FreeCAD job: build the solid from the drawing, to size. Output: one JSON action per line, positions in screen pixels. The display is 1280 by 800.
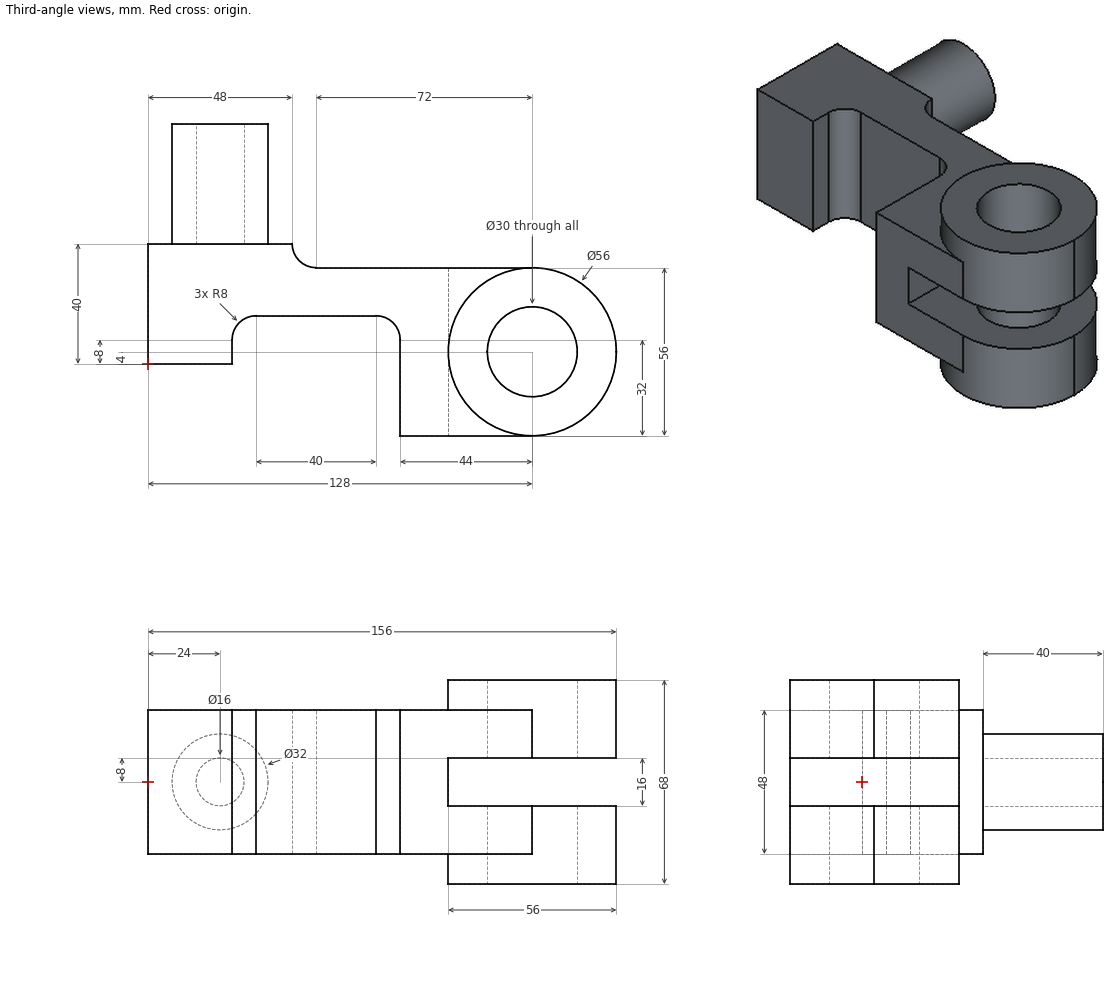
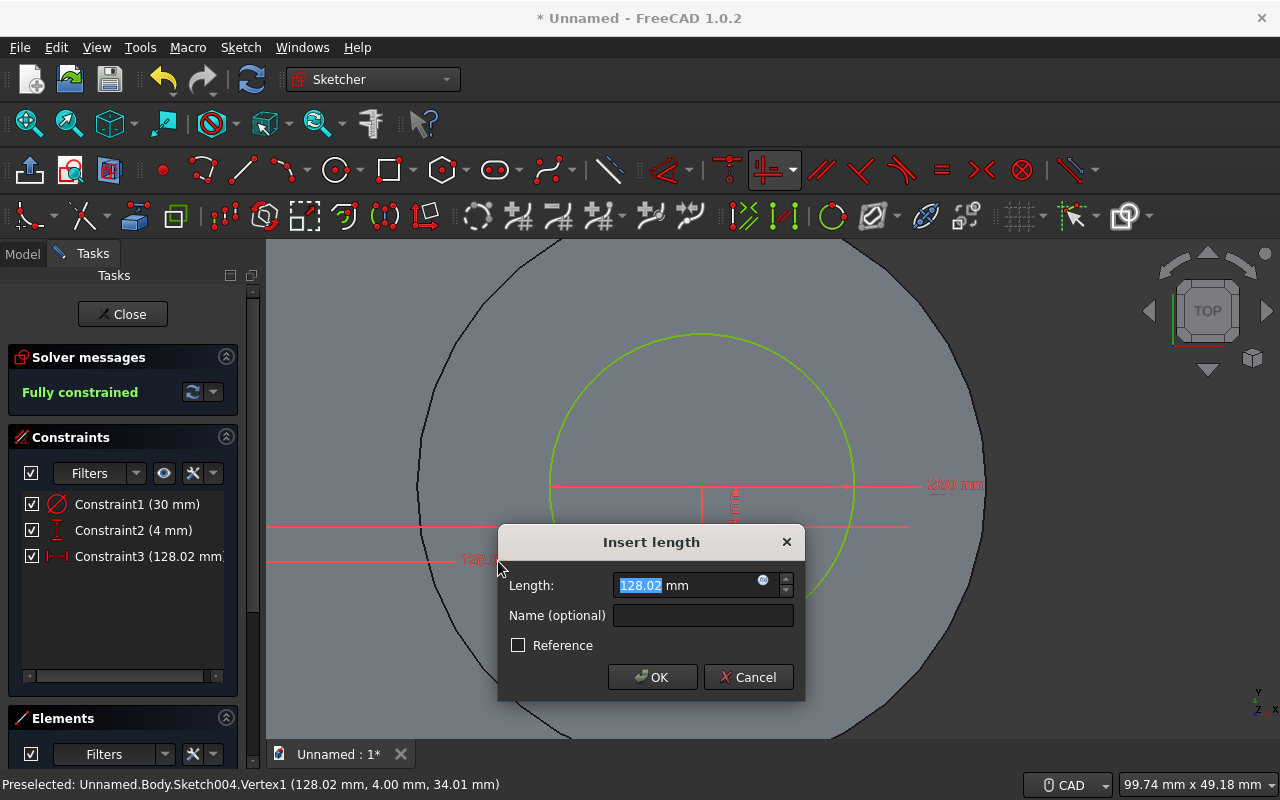
{"action": "type", "text": "128"}
{"action": "key", "text": "Return"}
{"action": "key", "text": "Escape"}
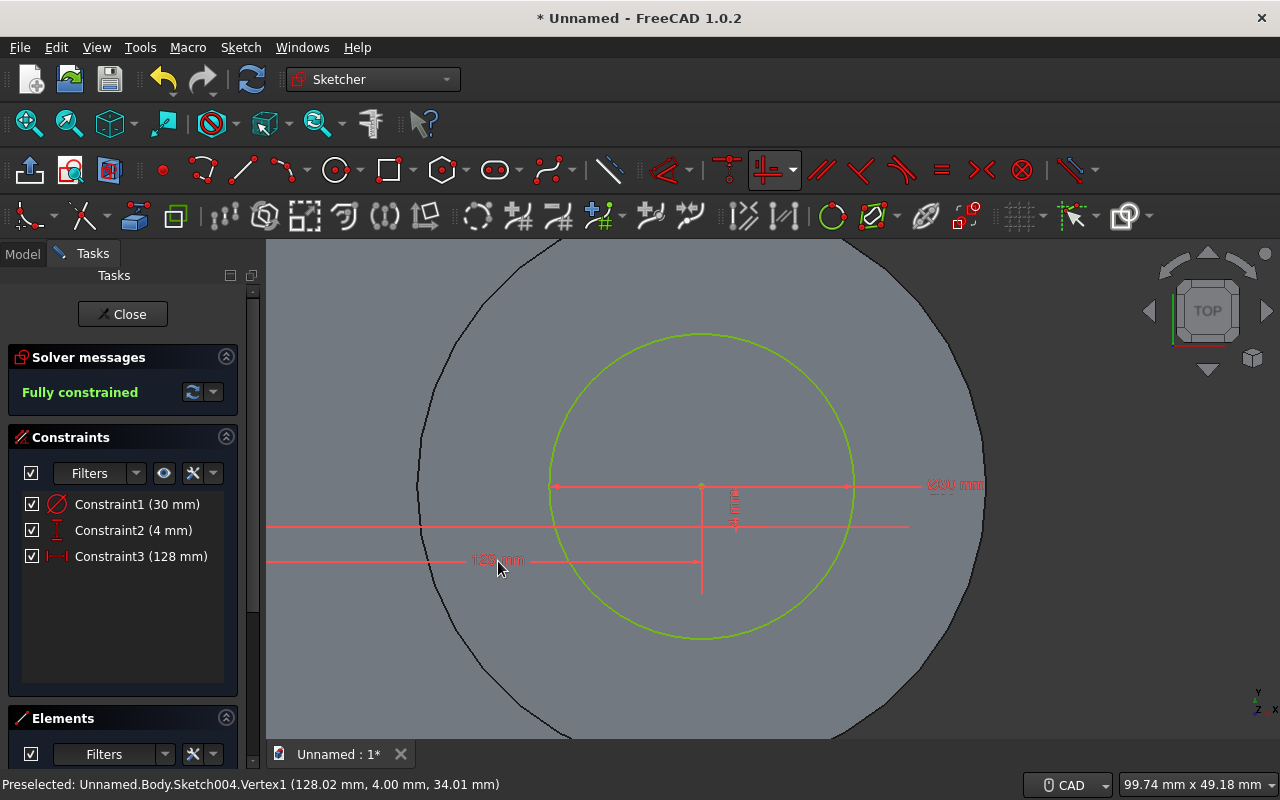
{"action": "left_click", "coordinate": [123, 314]}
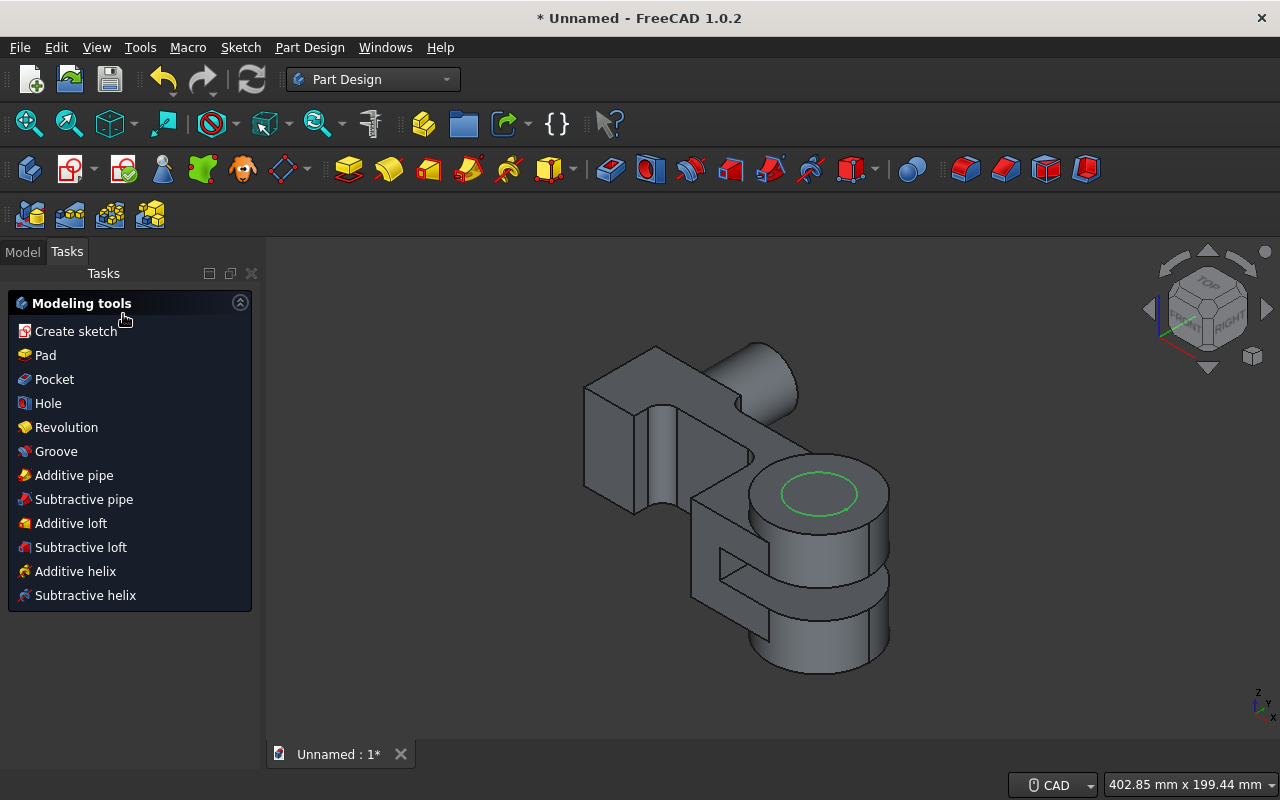
{"action": "left_click", "coordinate": [652, 170]}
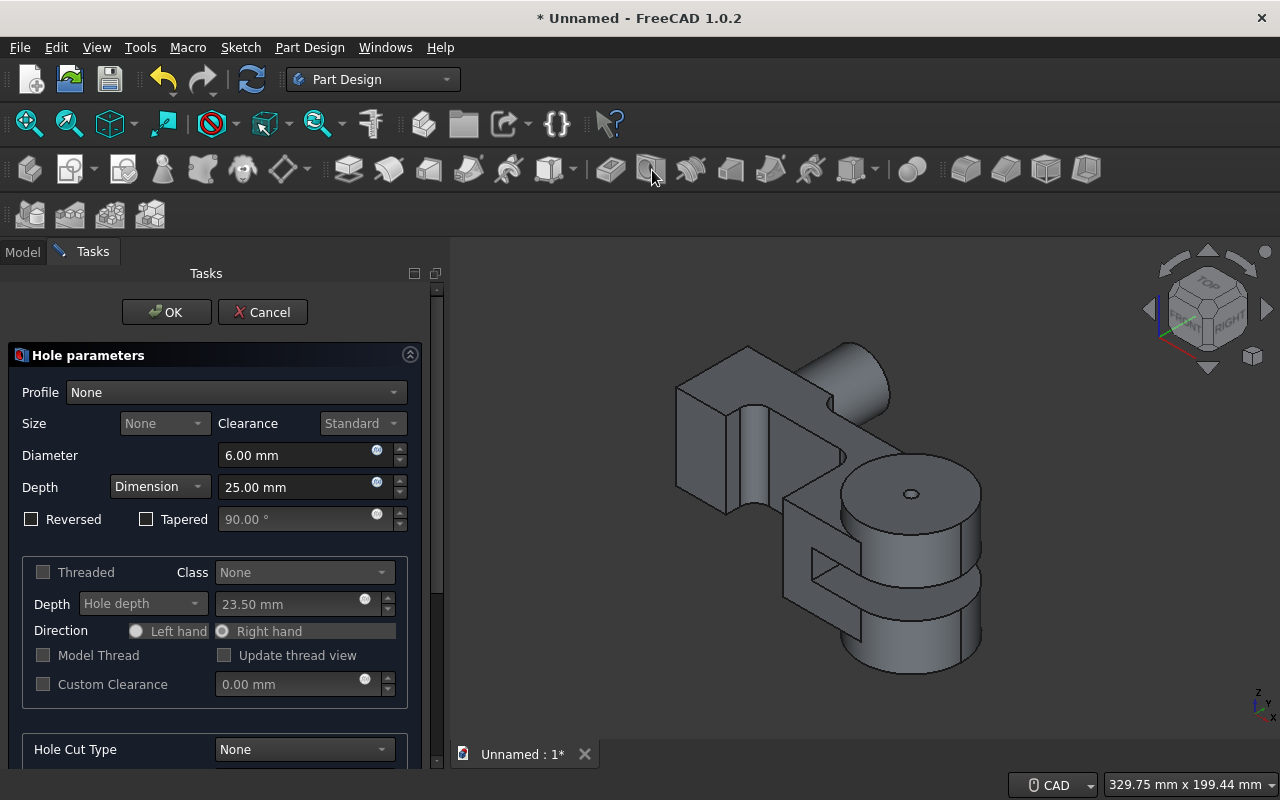
{"action": "triple_click", "coordinate": [305, 455]}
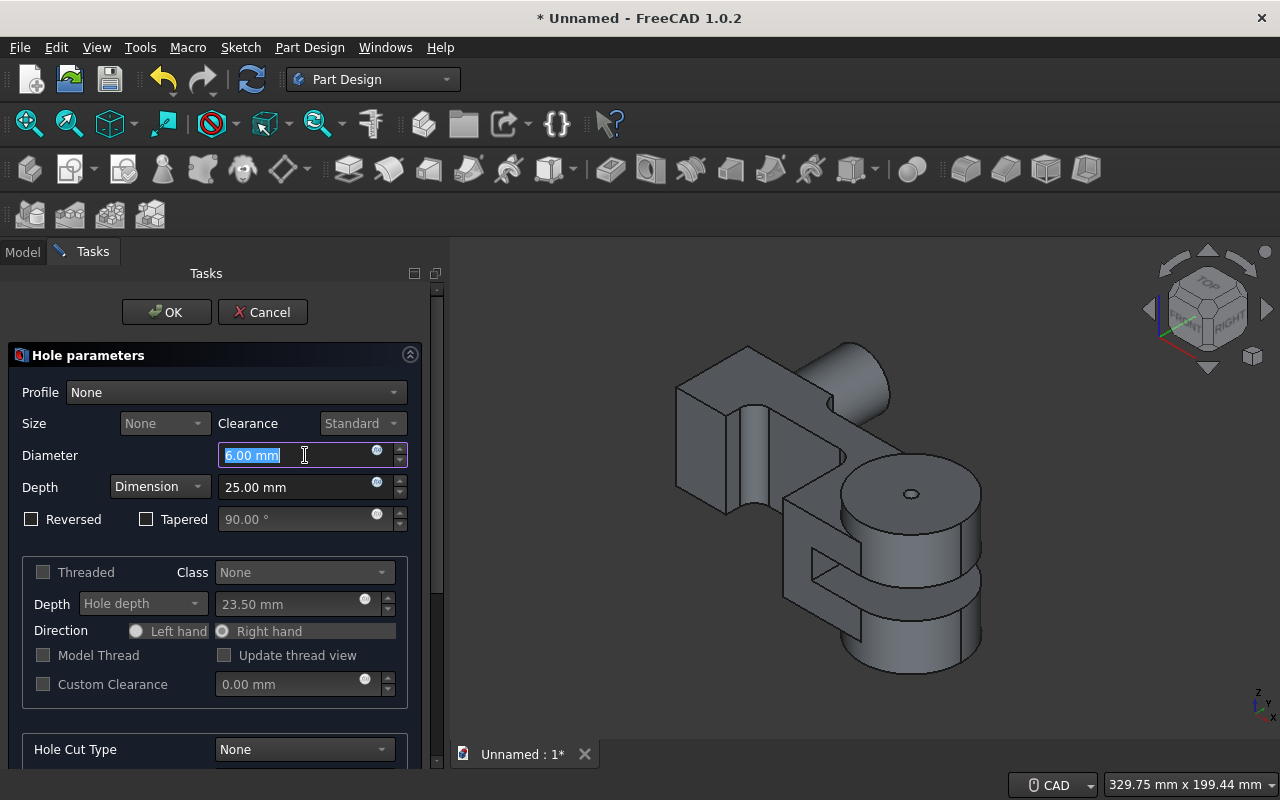
{"action": "type", "text": "30"}
{"action": "key", "text": "Tab"}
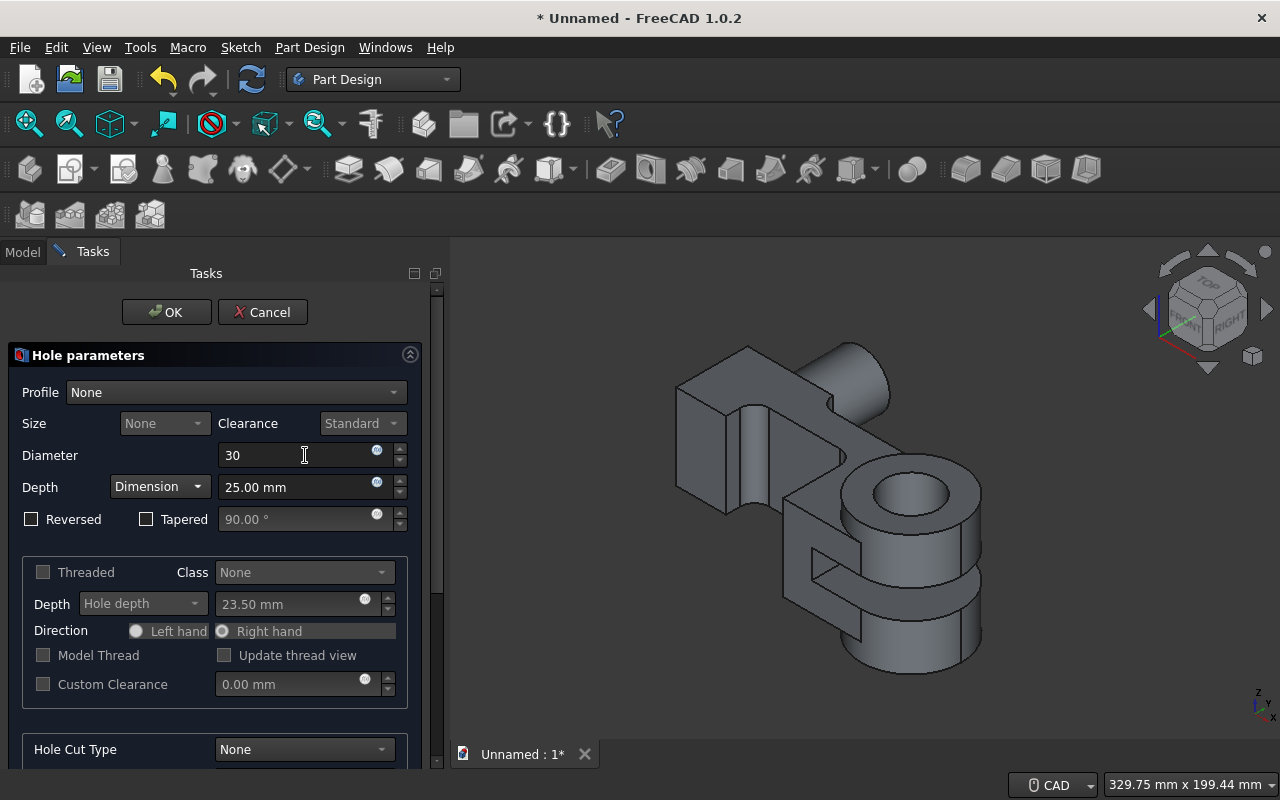
{"action": "left_click", "coordinate": [161, 486]}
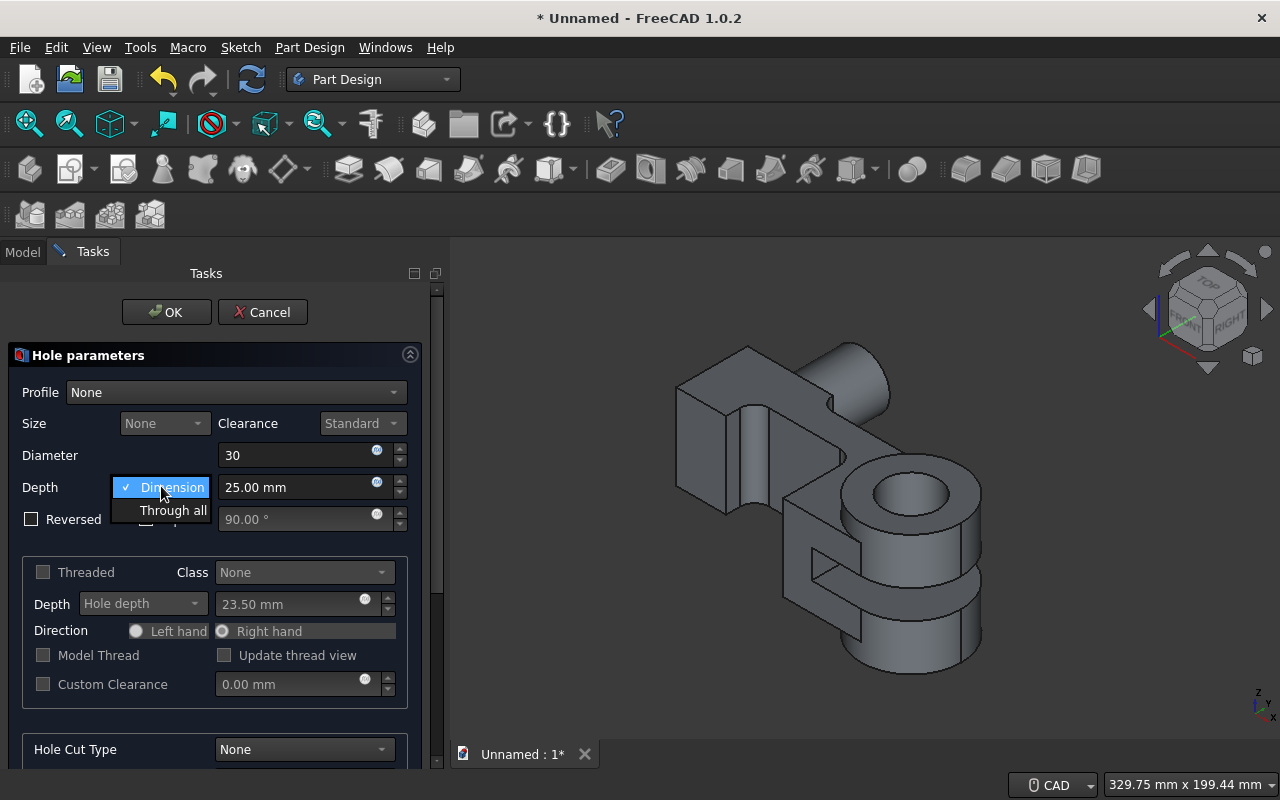
{"action": "left_click", "coordinate": [160, 510]}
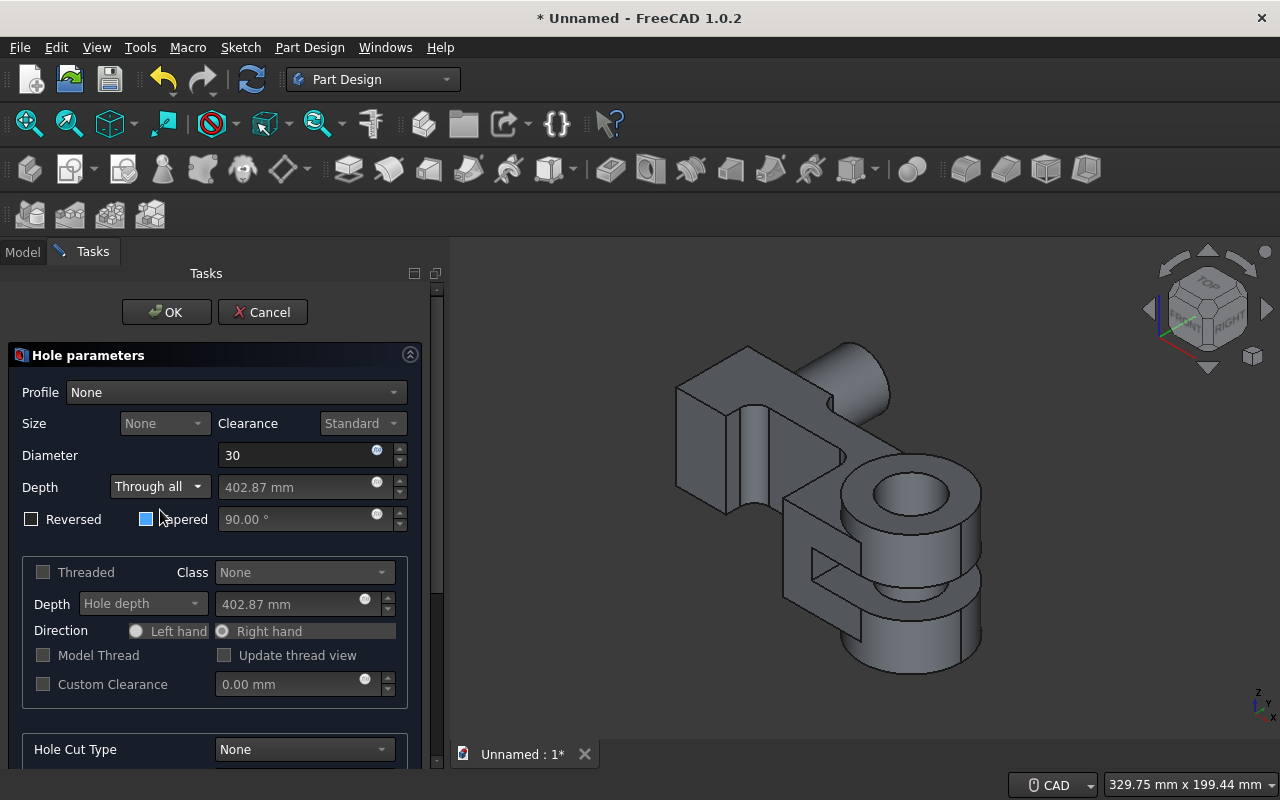
{"action": "left_click", "coordinate": [167, 312]}